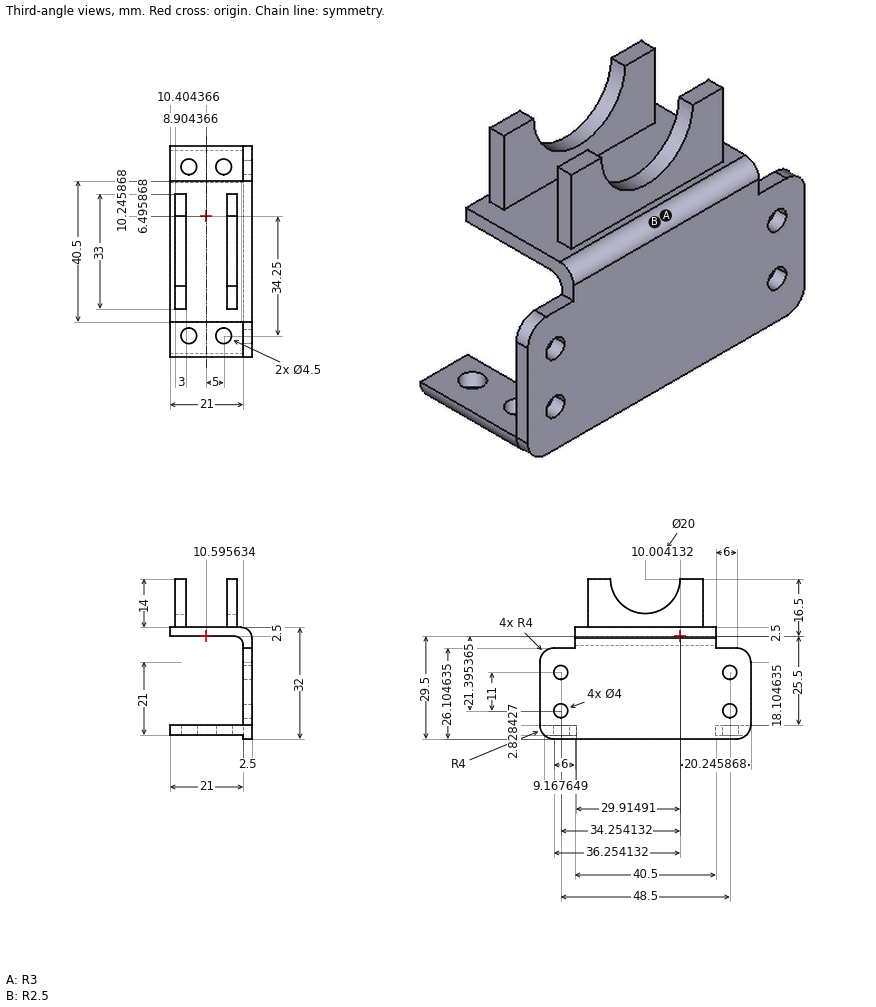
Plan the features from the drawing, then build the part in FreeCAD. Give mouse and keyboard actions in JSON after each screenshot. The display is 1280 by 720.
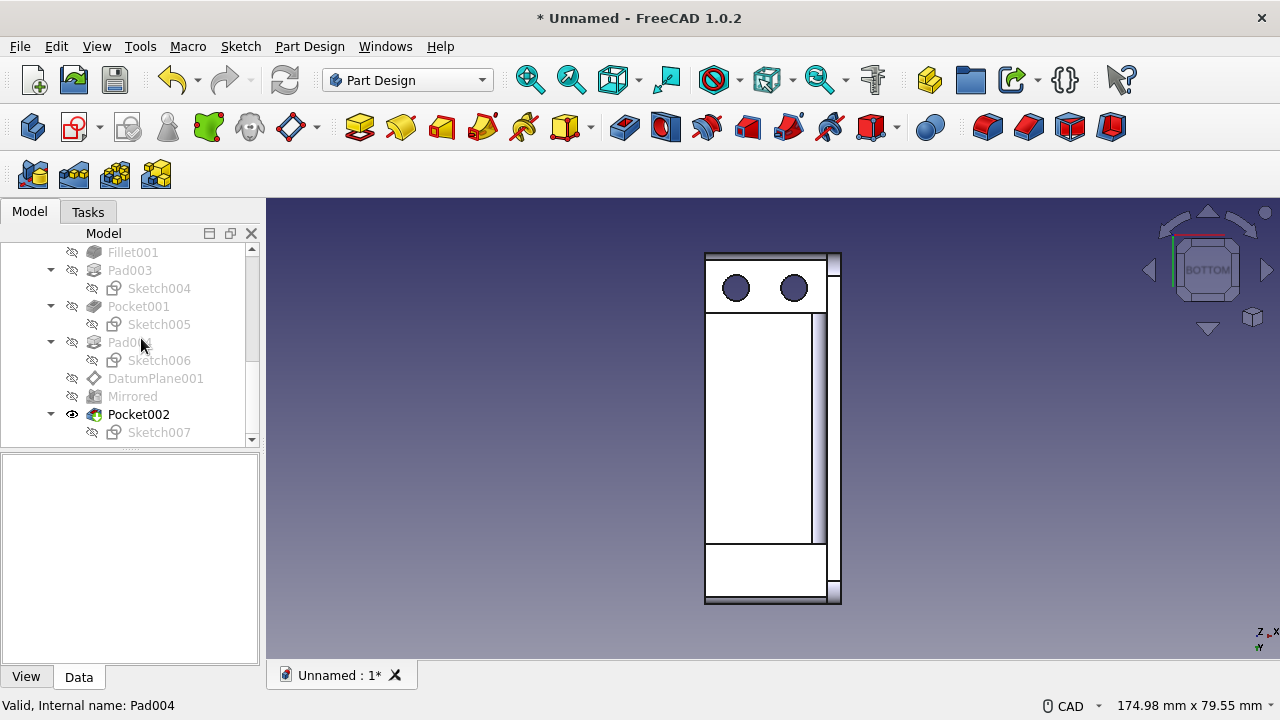
{"action": "scroll", "coordinate": [141, 338], "scroll_direction": "up", "scroll_amount": 15}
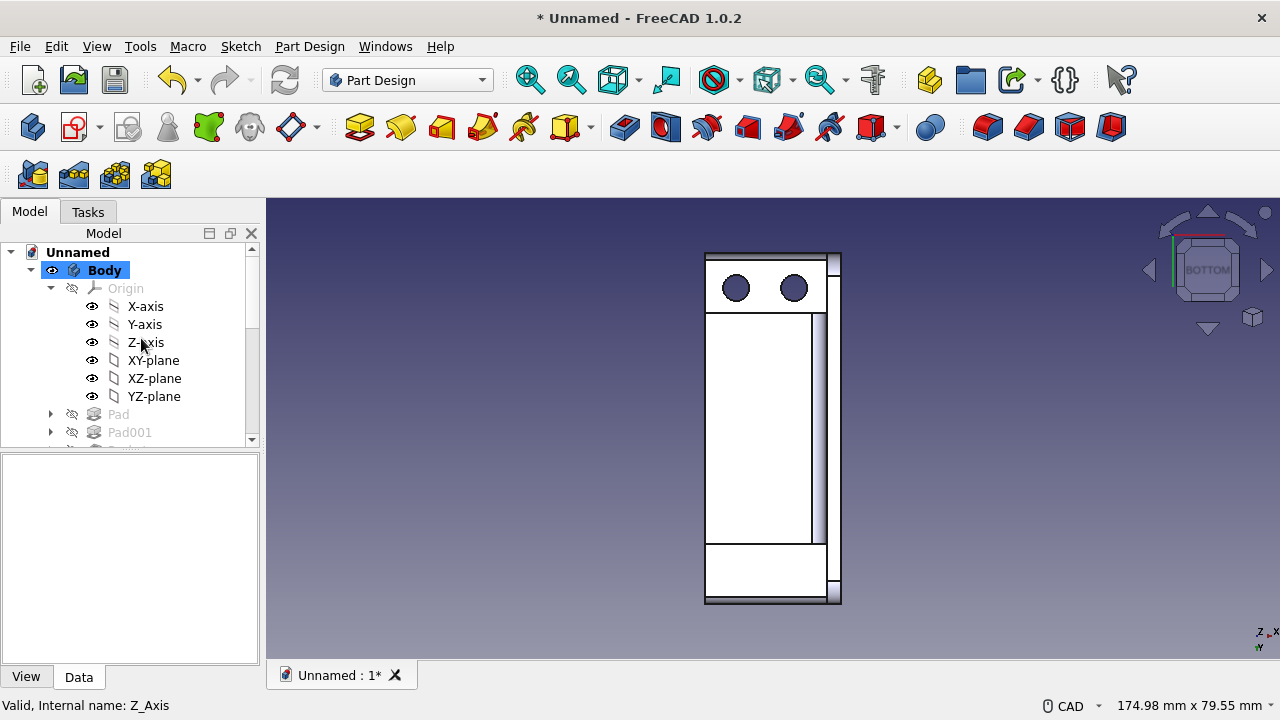
{"action": "left_click", "coordinate": [137, 378]}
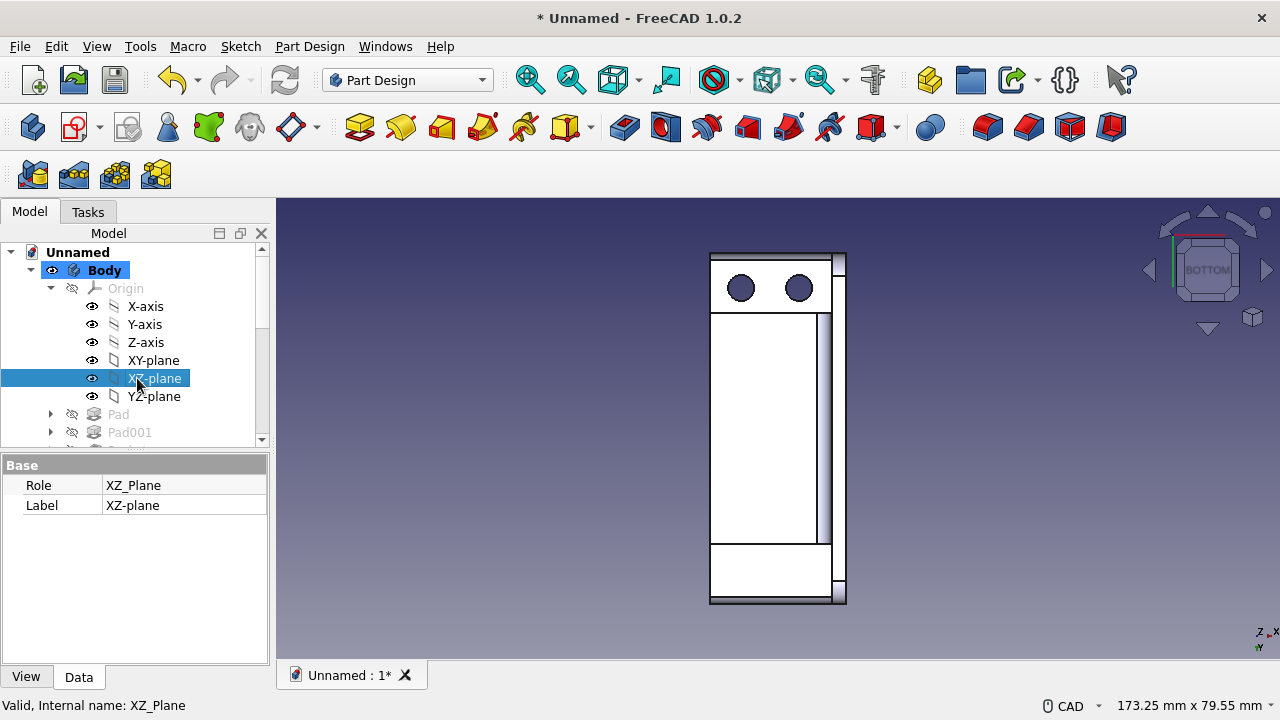
{"action": "left_click", "coordinate": [290, 128]}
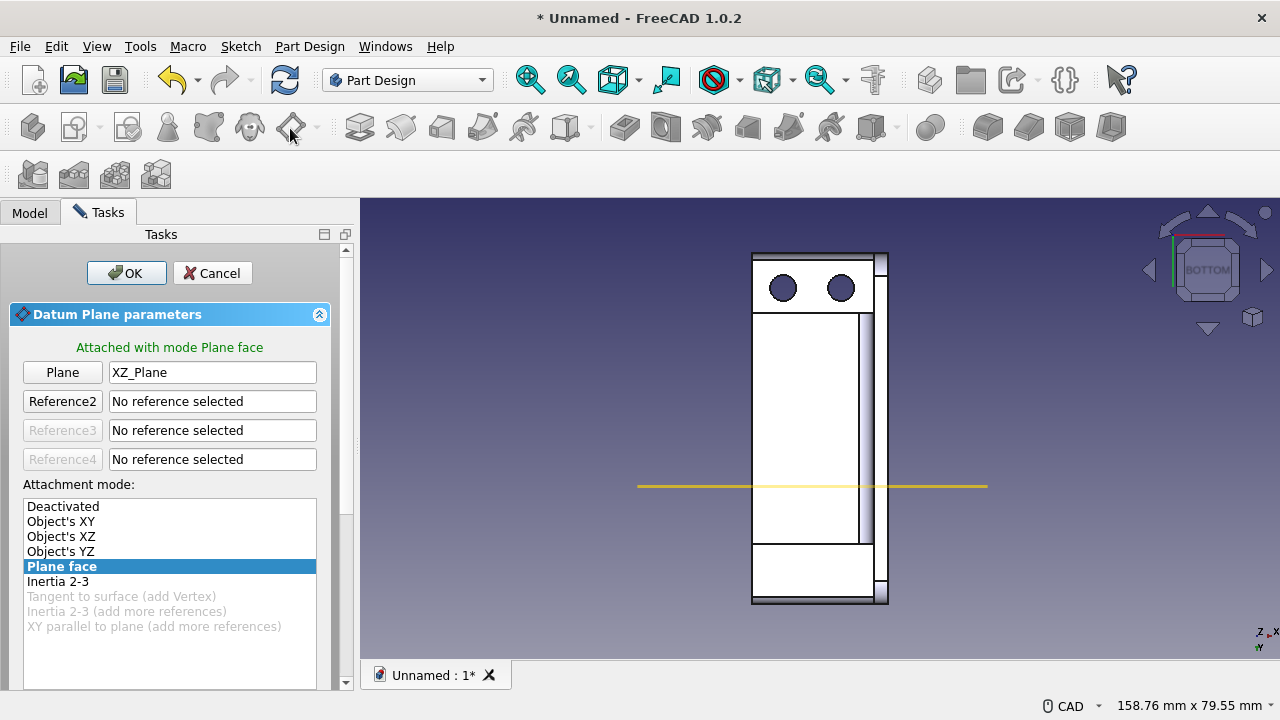
{"action": "scroll", "coordinate": [346, 467], "scroll_direction": "down", "scroll_amount": 4}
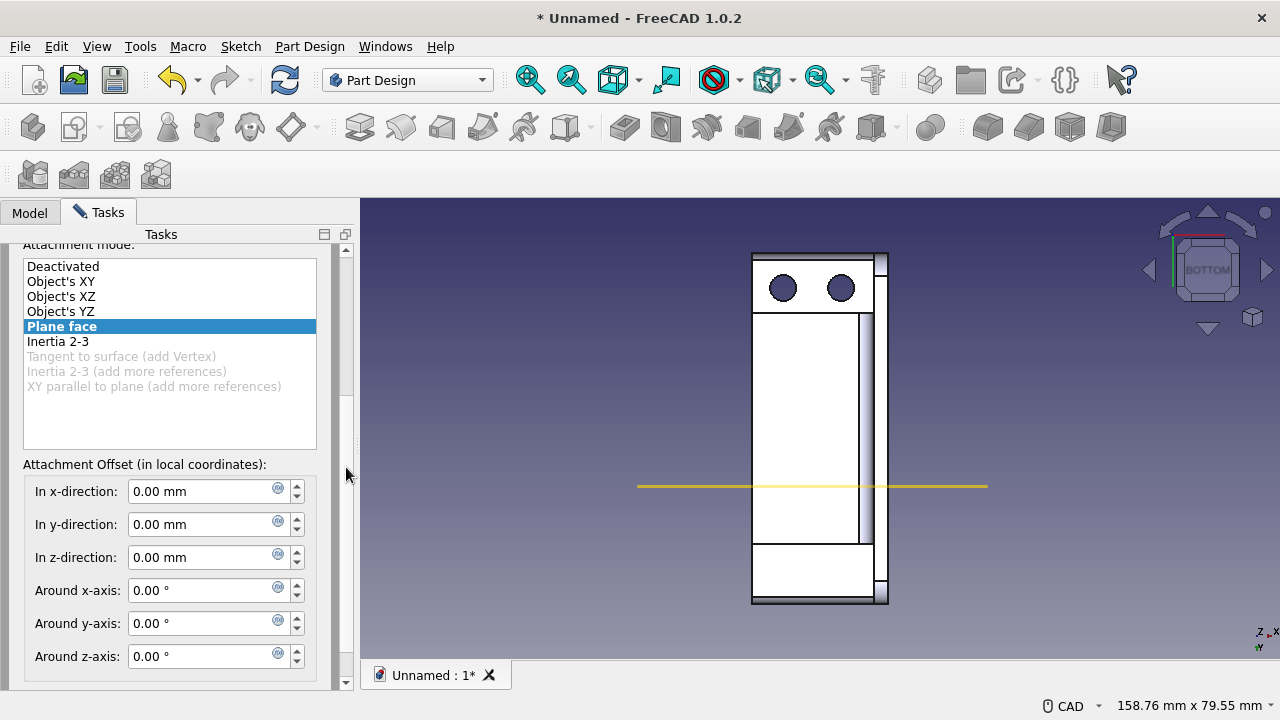
{"action": "triple_click", "coordinate": [210, 558]}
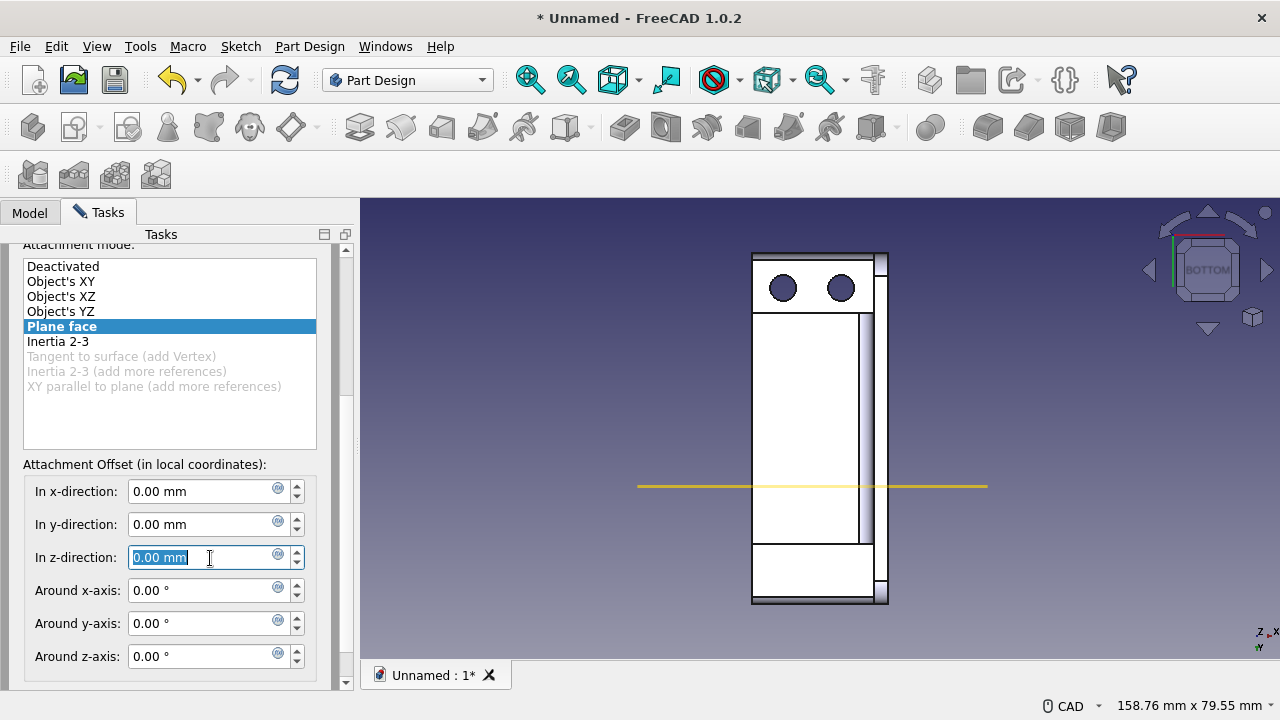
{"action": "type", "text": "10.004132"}
{"action": "key", "text": "Tab"}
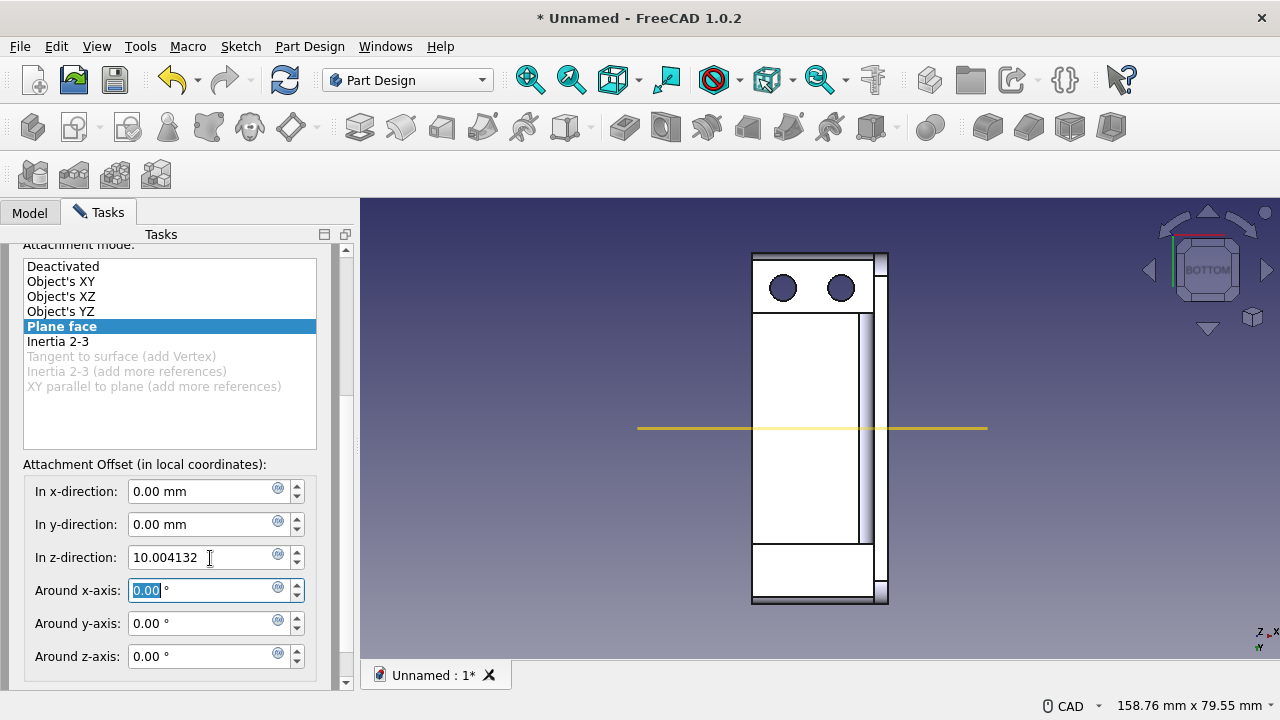
{"action": "scroll", "coordinate": [346, 467], "scroll_direction": "up", "scroll_amount": 5}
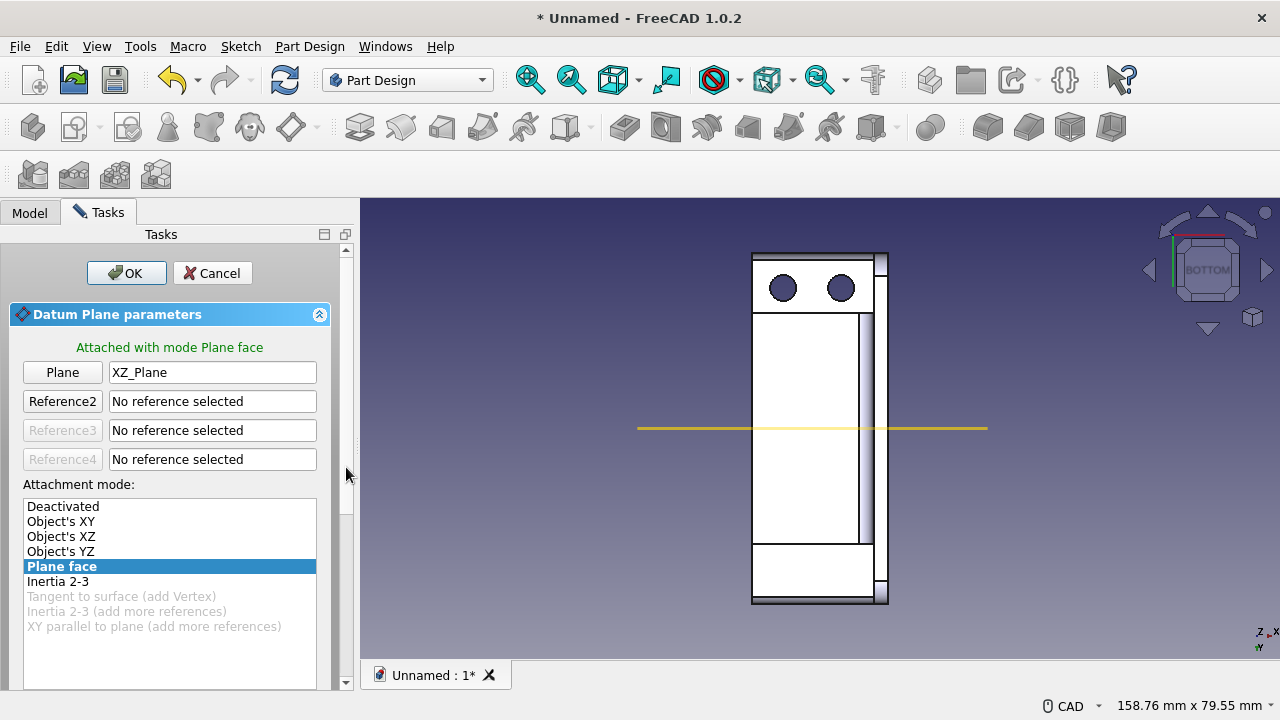
{"action": "left_click", "coordinate": [127, 273]}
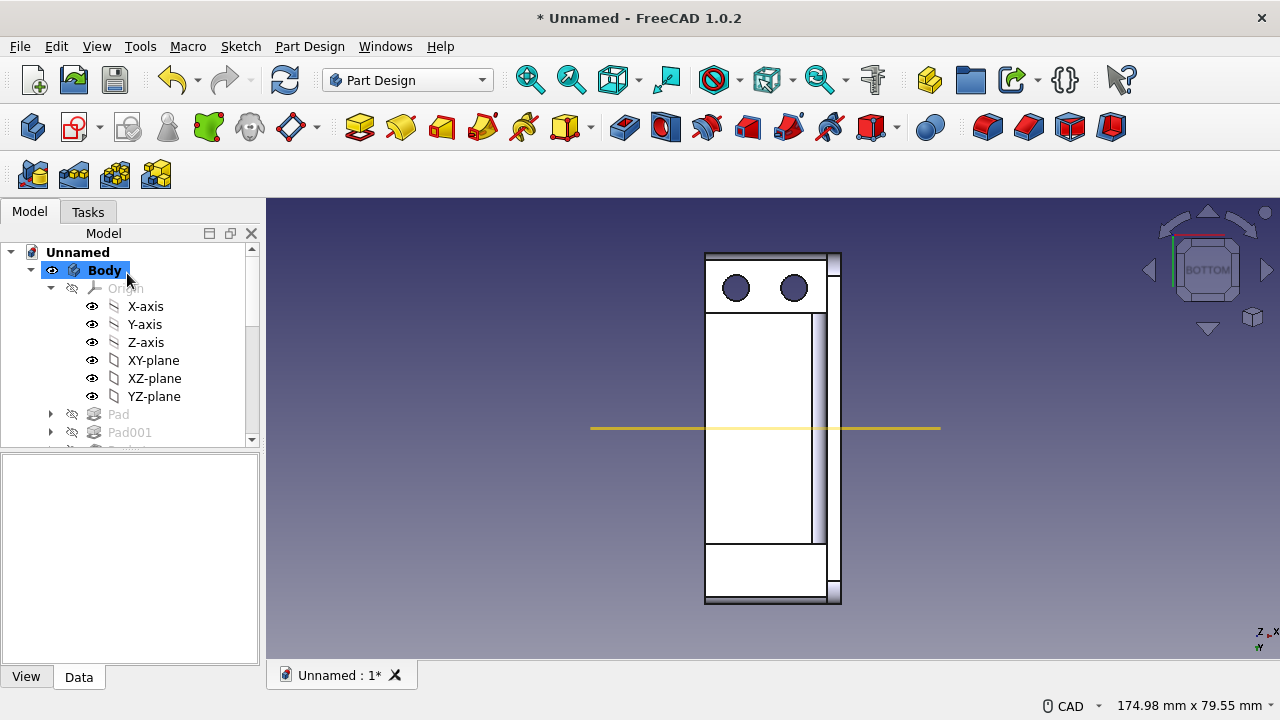
{"action": "scroll", "coordinate": [101, 338], "scroll_direction": "down", "scroll_amount": 3}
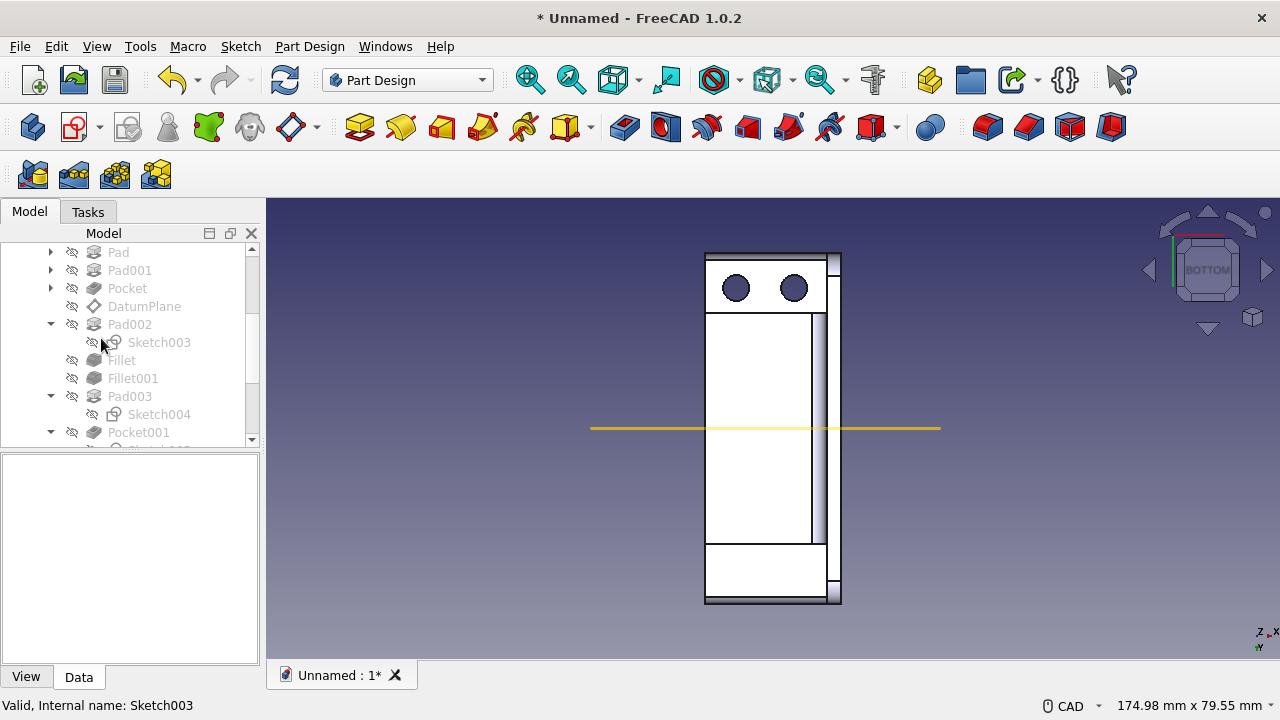
{"action": "scroll", "coordinate": [141, 338], "scroll_direction": "up", "scroll_amount": 15}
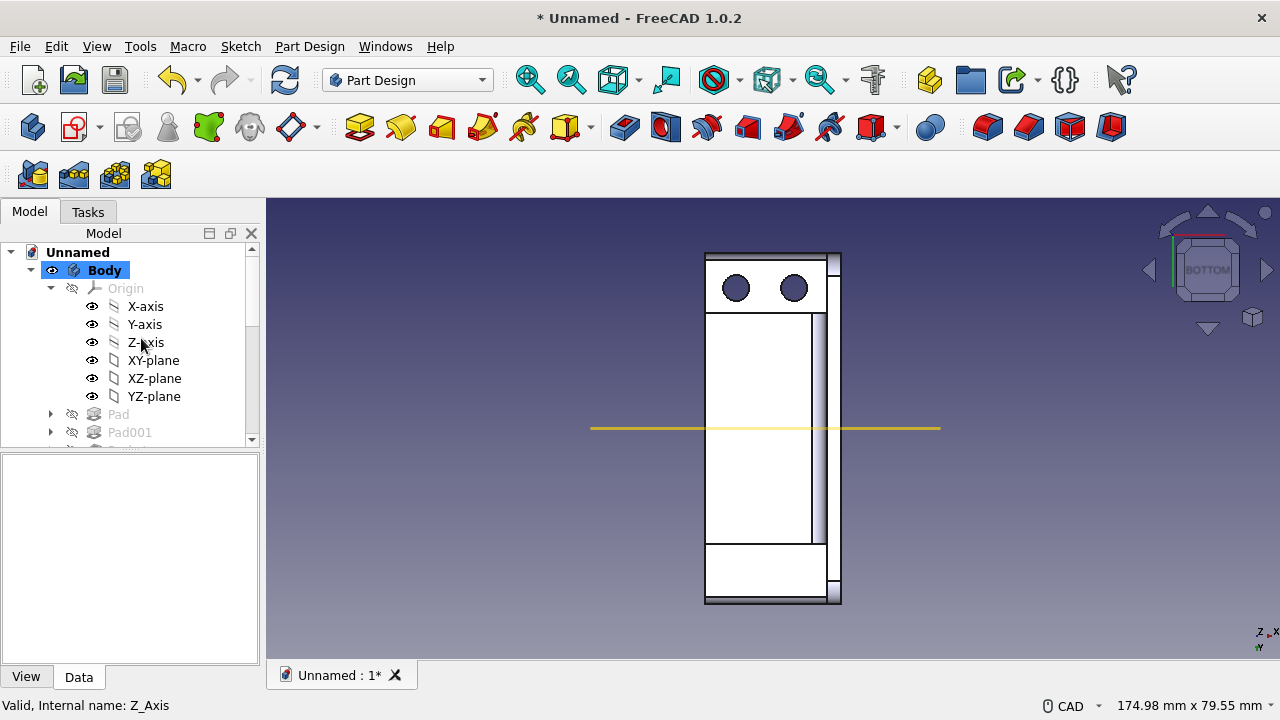
{"action": "scroll", "coordinate": [101, 338], "scroll_direction": "down", "scroll_amount": 6}